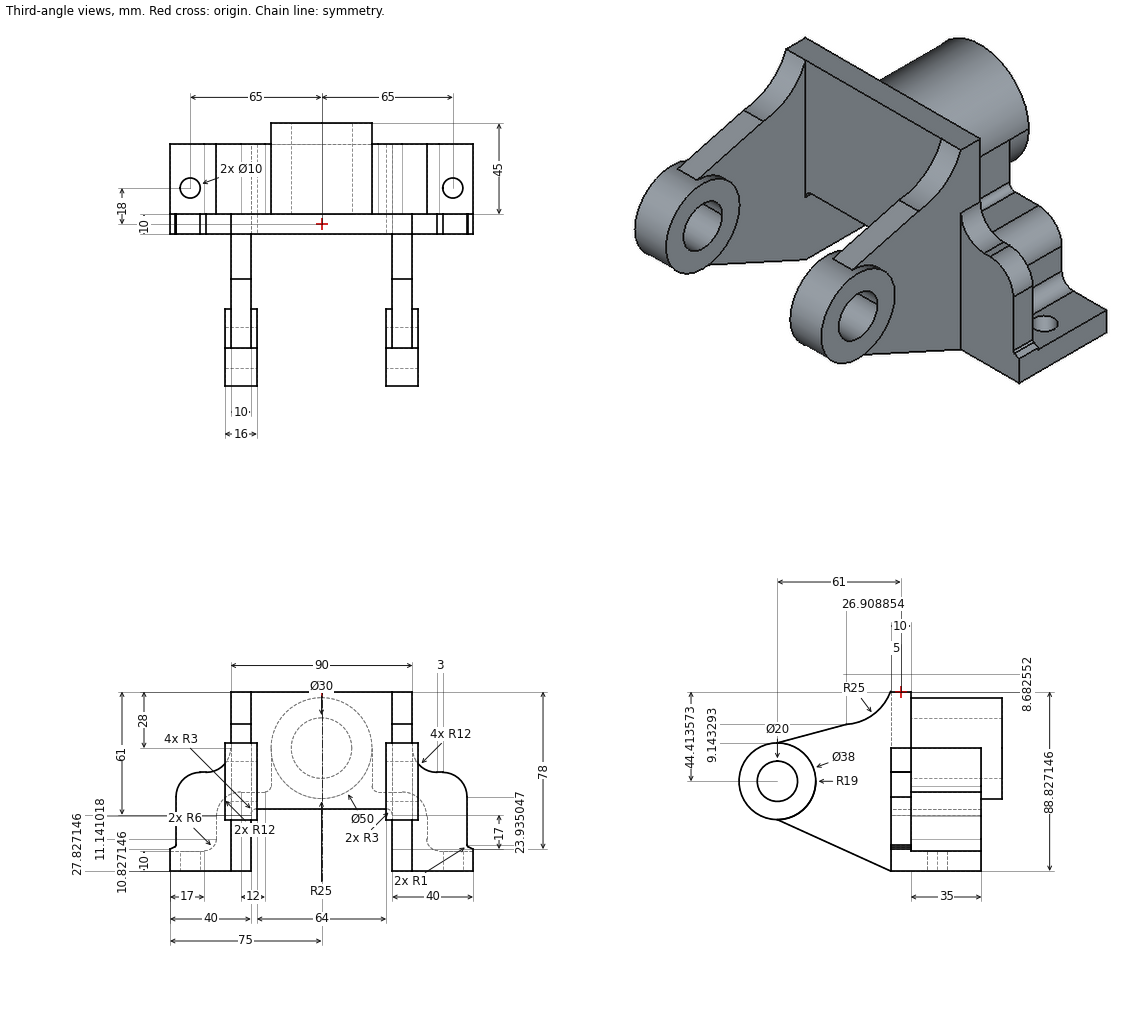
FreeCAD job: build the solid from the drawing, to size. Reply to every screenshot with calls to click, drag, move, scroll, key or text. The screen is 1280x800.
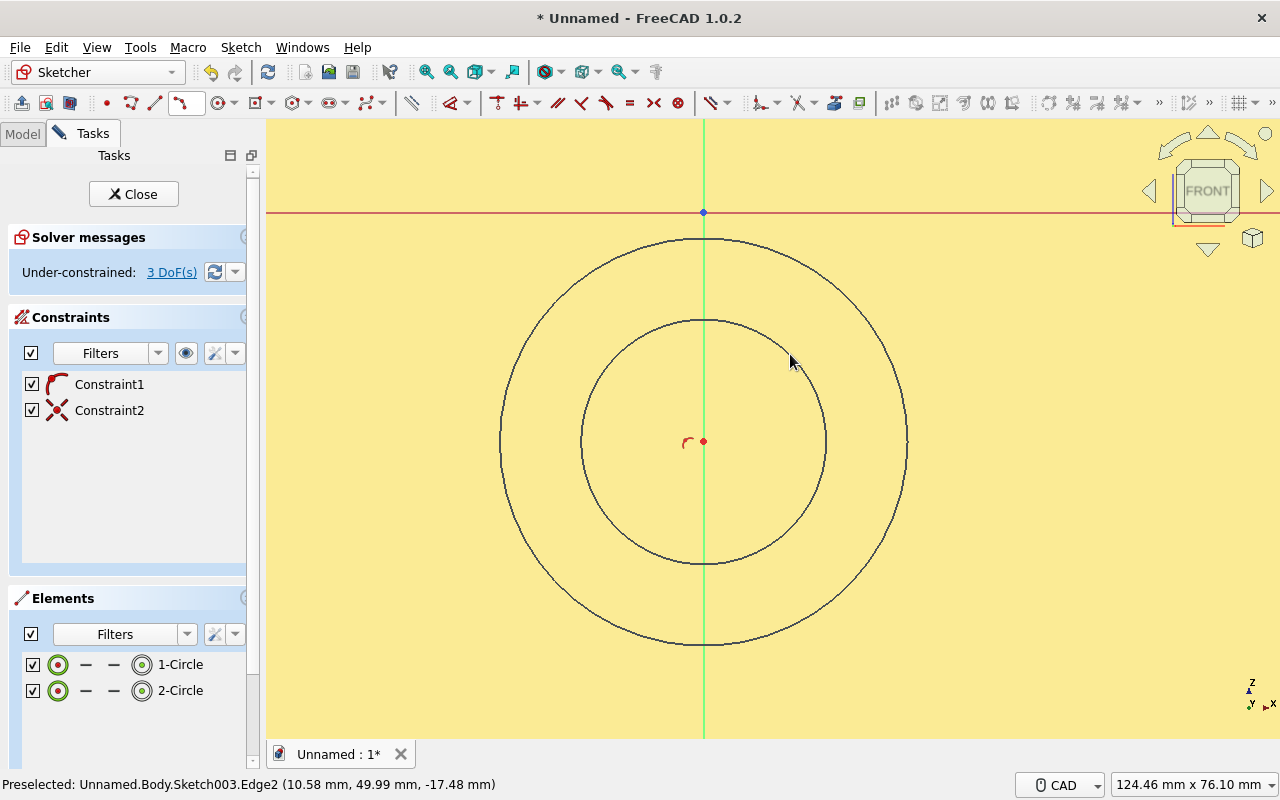
key(d)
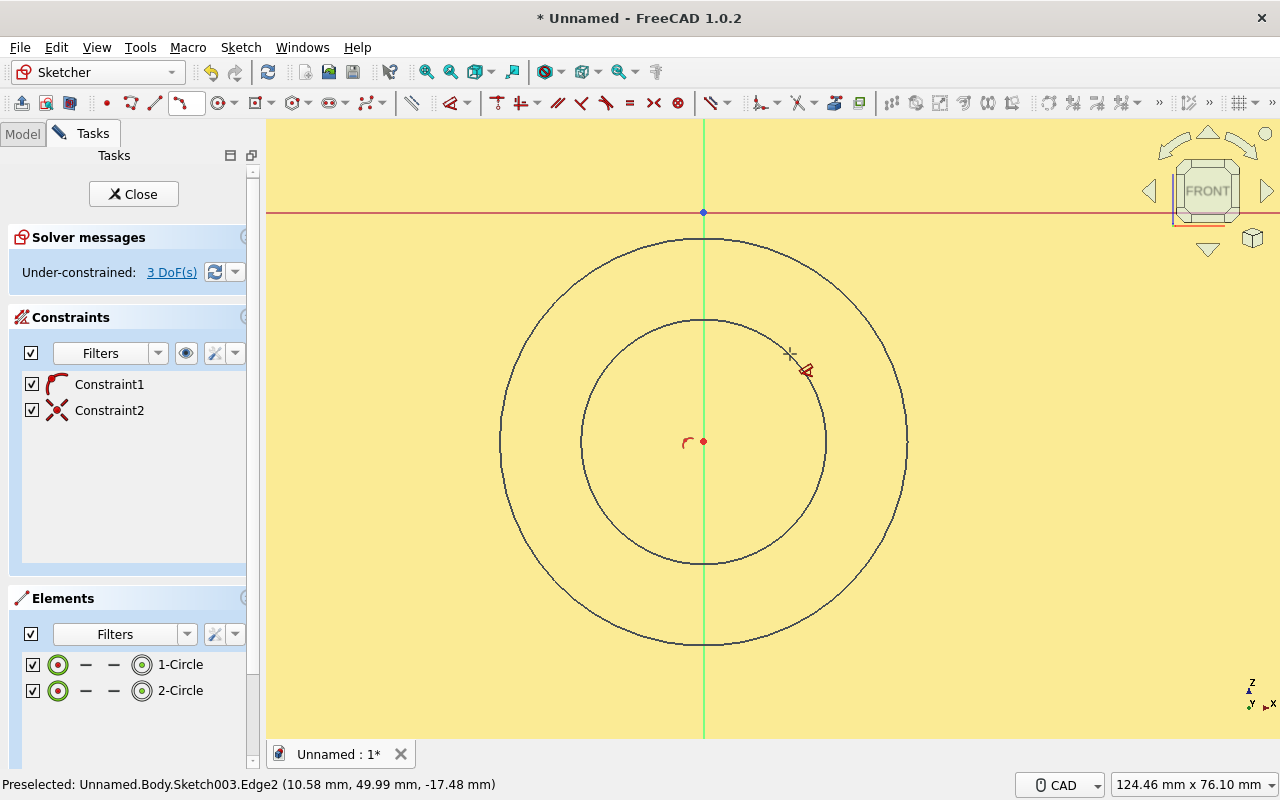
click(847, 297)
click(869, 274)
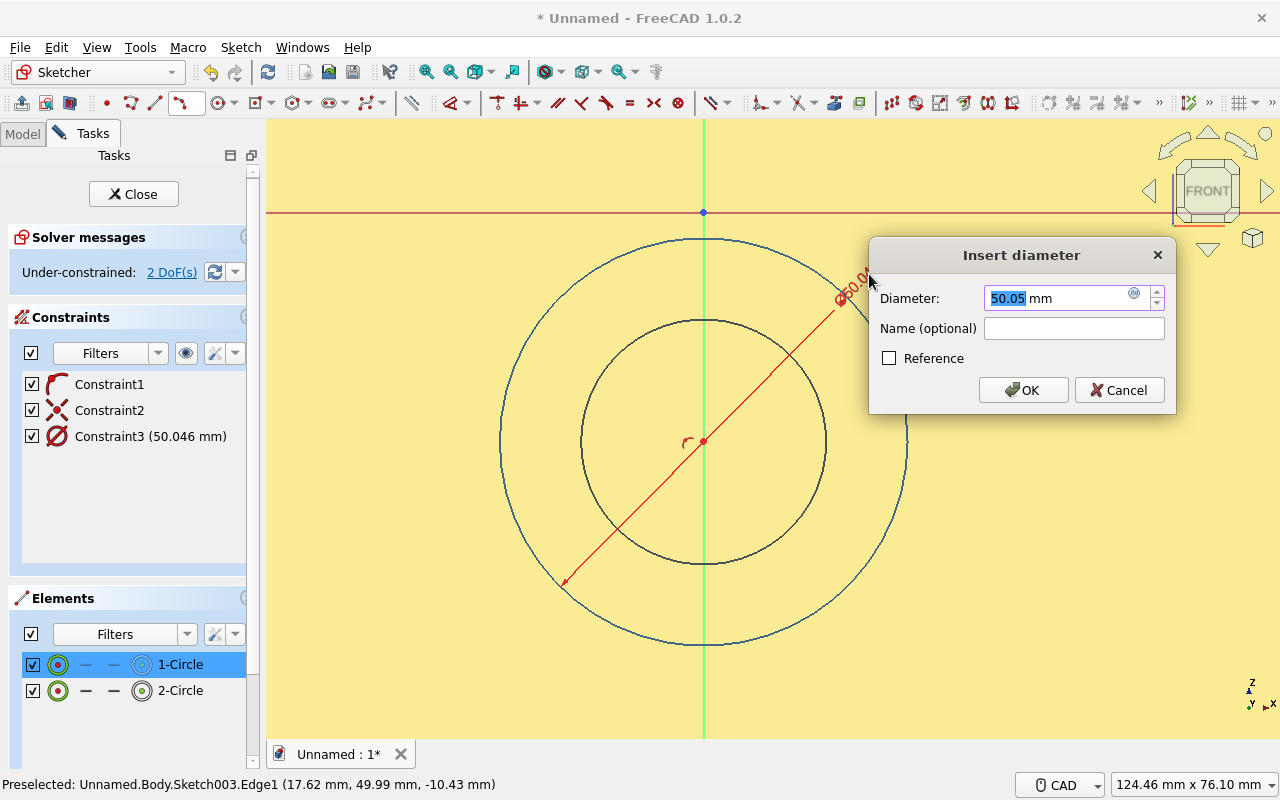
text(50)
key(Return)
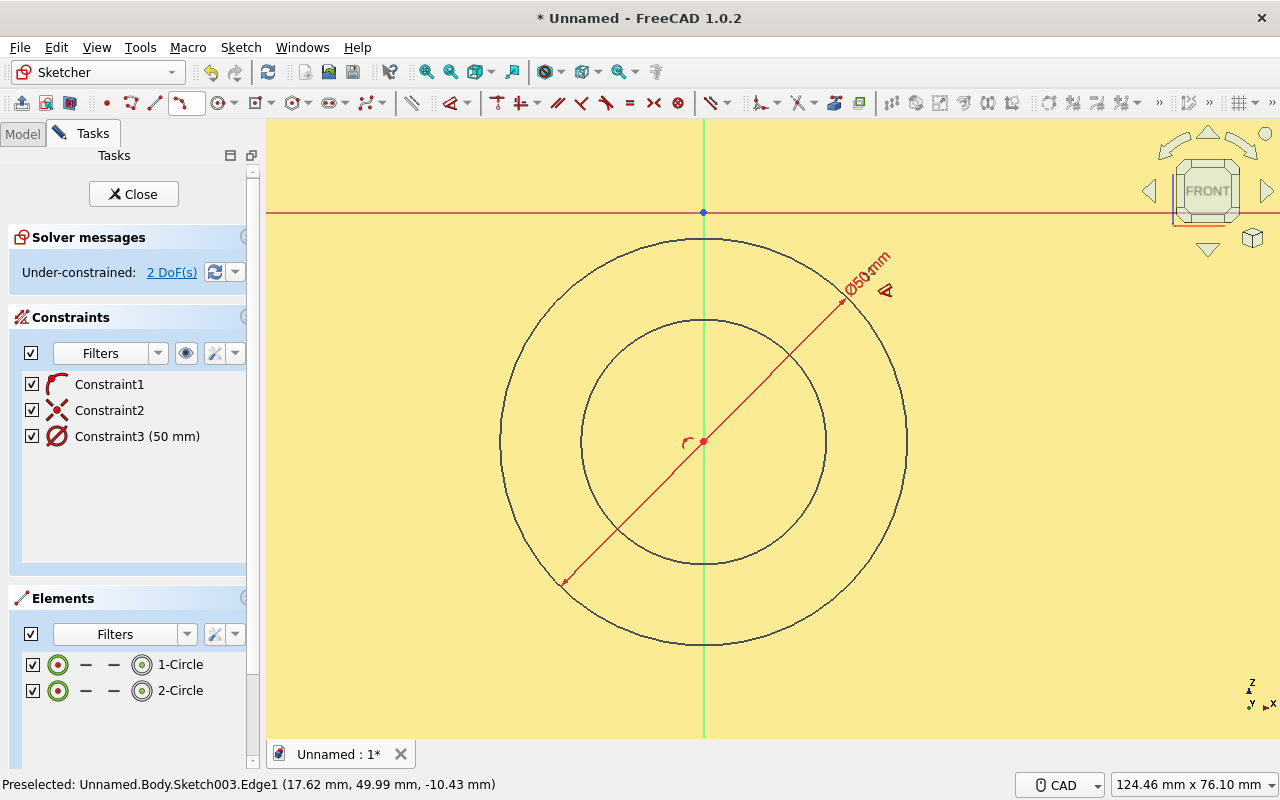
click(790, 355)
click(813, 332)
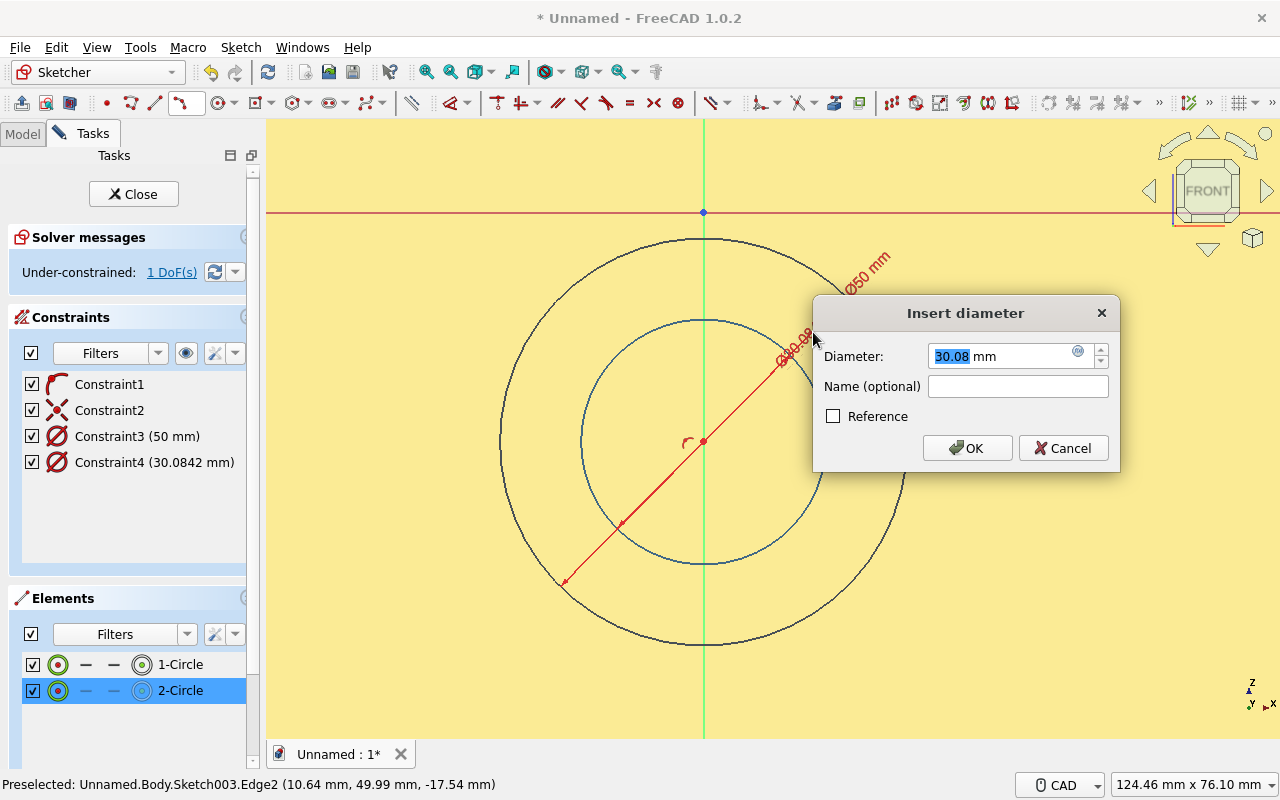
text(30)
key(Return)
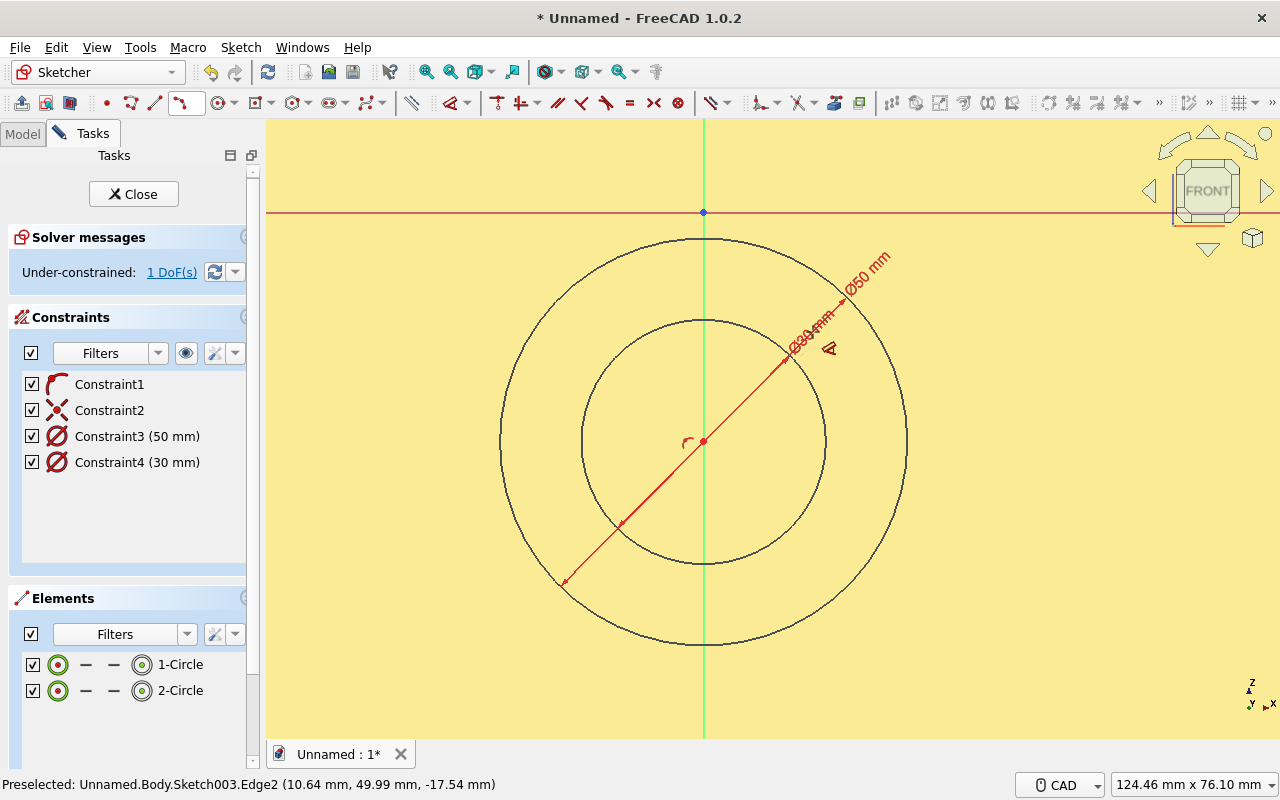
click(704, 442)
click(738, 275)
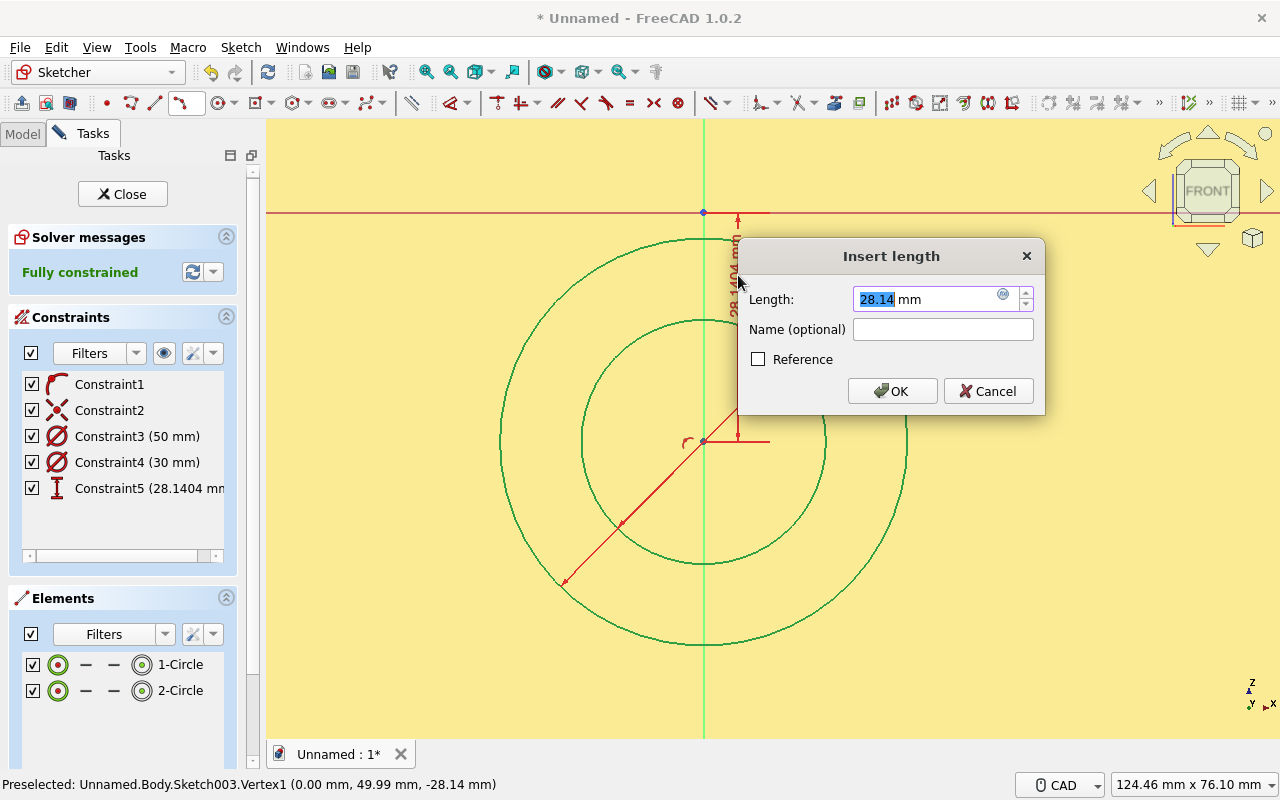
text(28)
key(Return)
key(Escape)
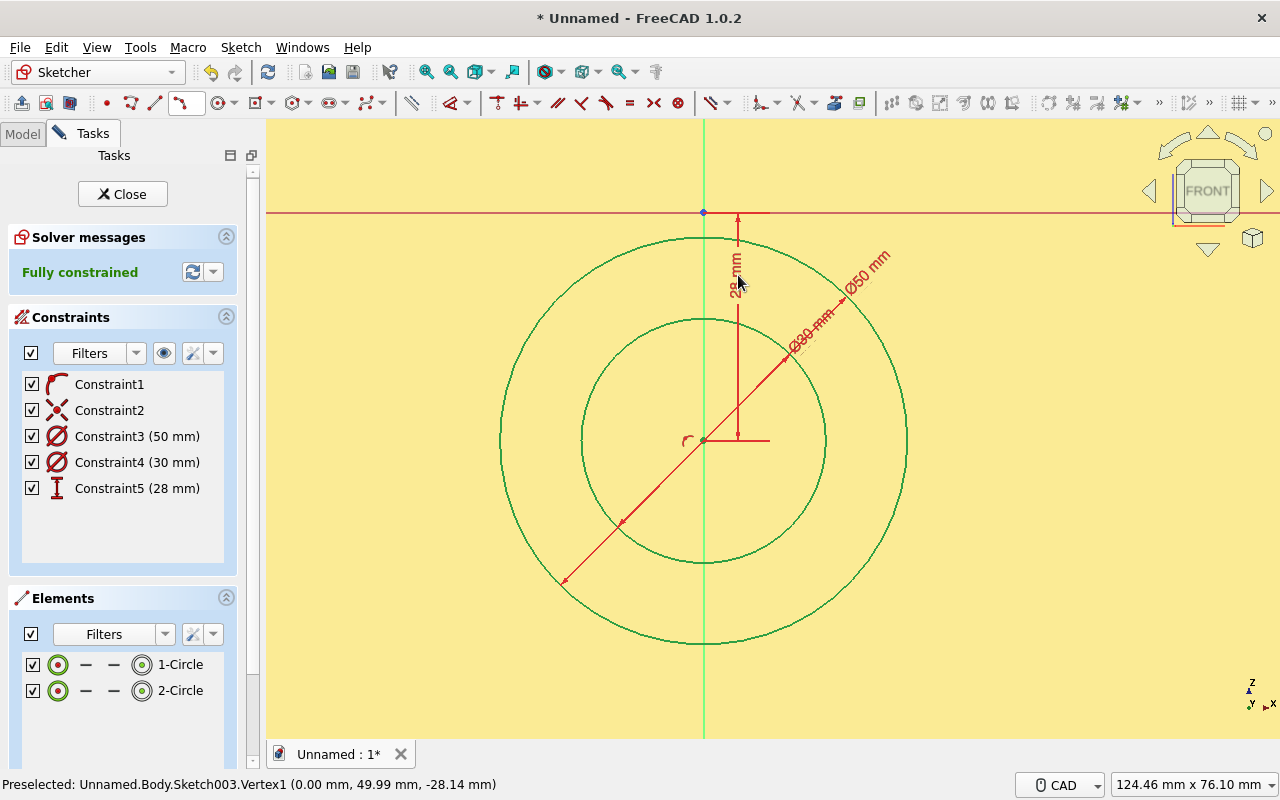
click(123, 194)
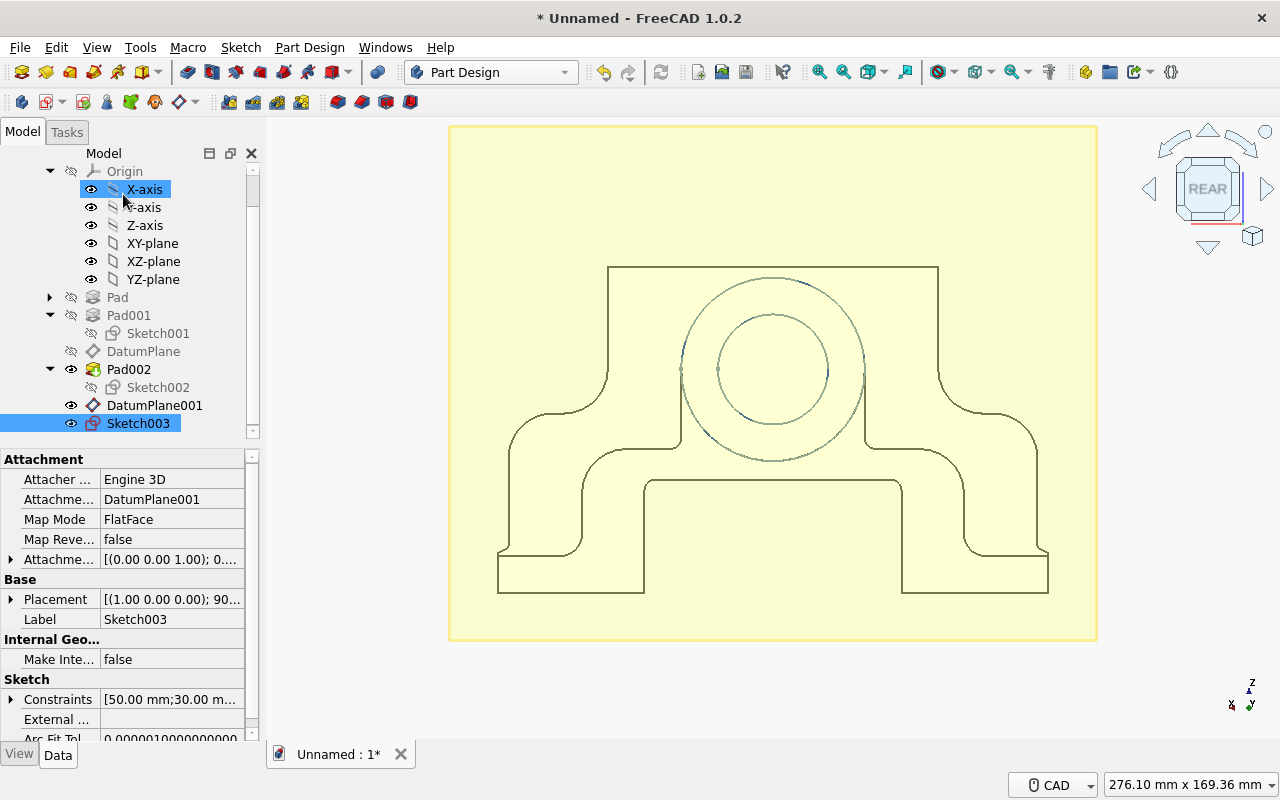
click(22, 72)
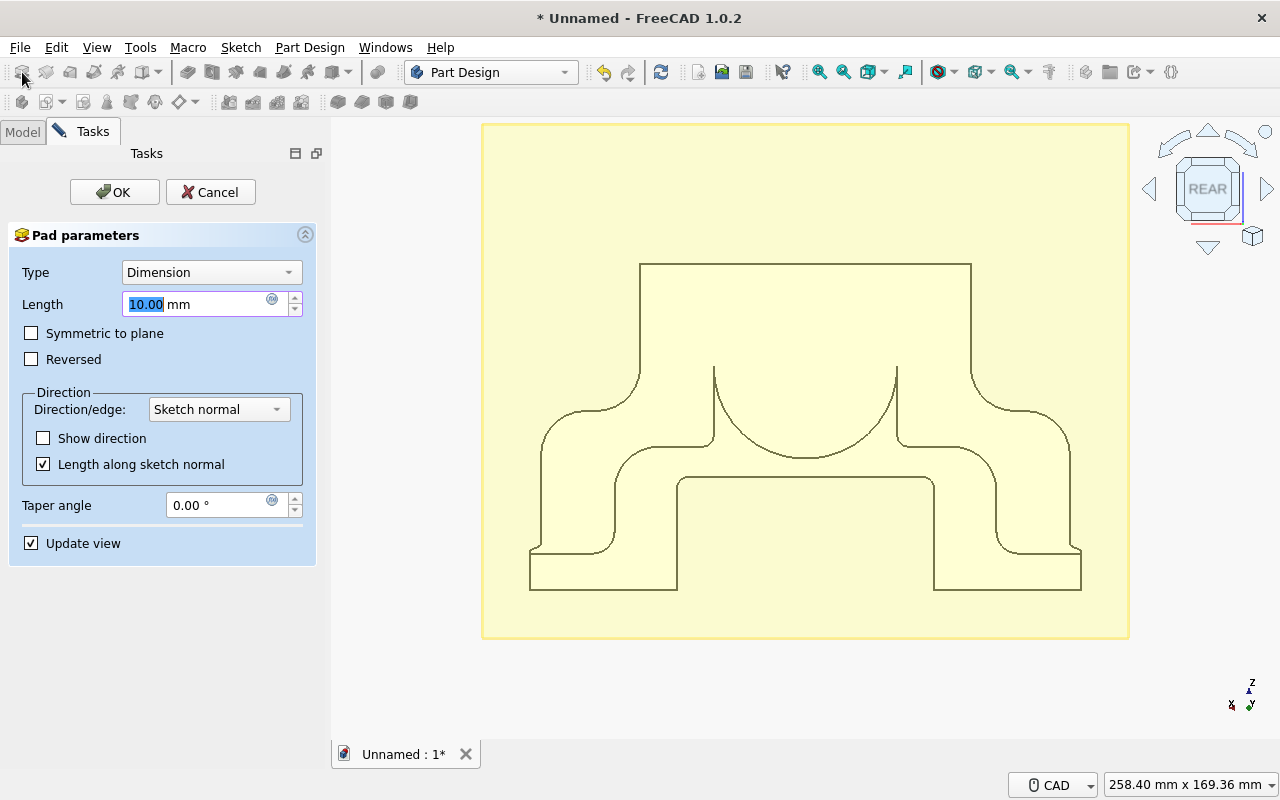
text(45)
key(Tab)